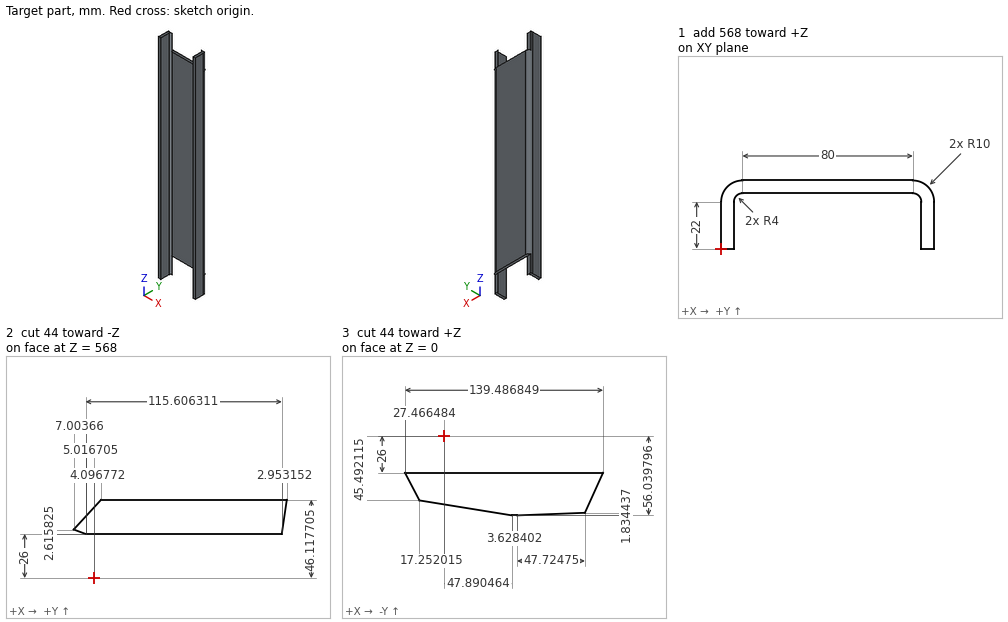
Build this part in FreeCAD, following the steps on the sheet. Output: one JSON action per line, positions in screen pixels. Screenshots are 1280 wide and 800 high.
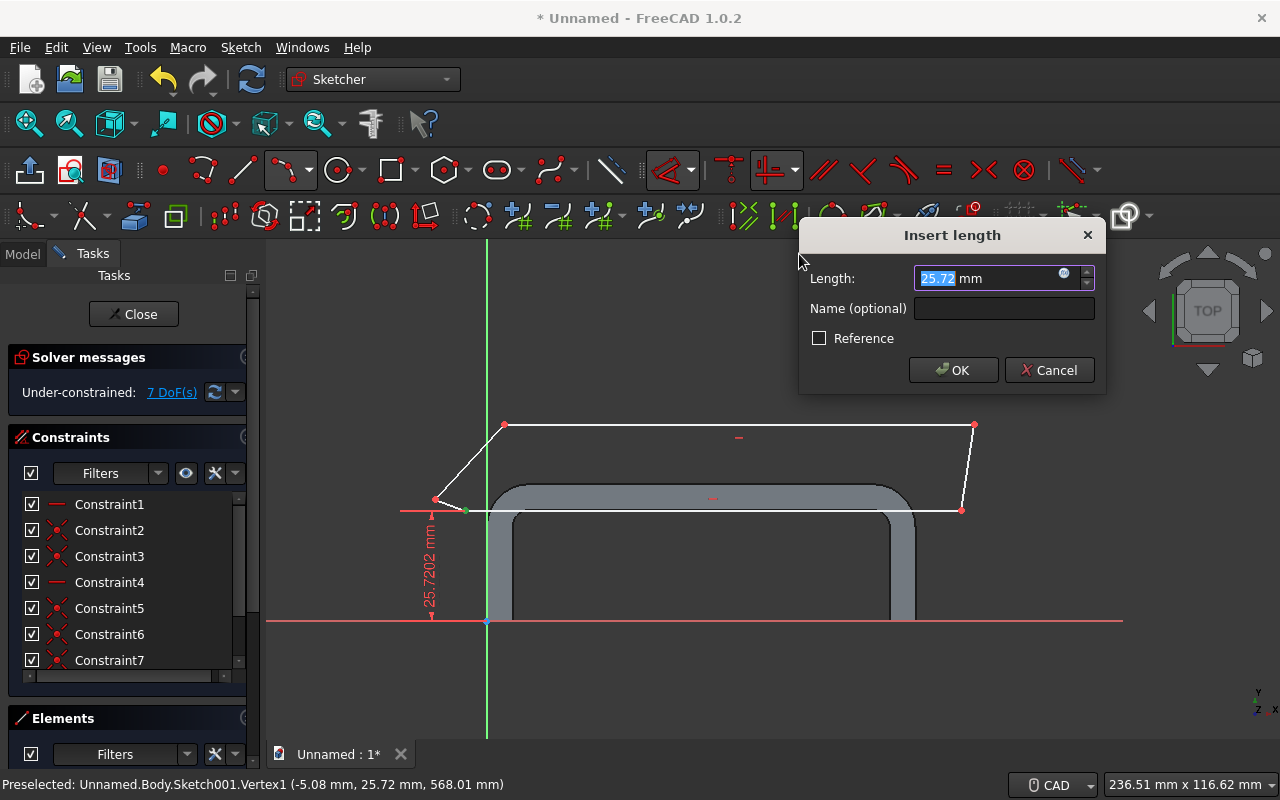
{"action": "type", "text": "26"}
{"action": "key", "text": "Return"}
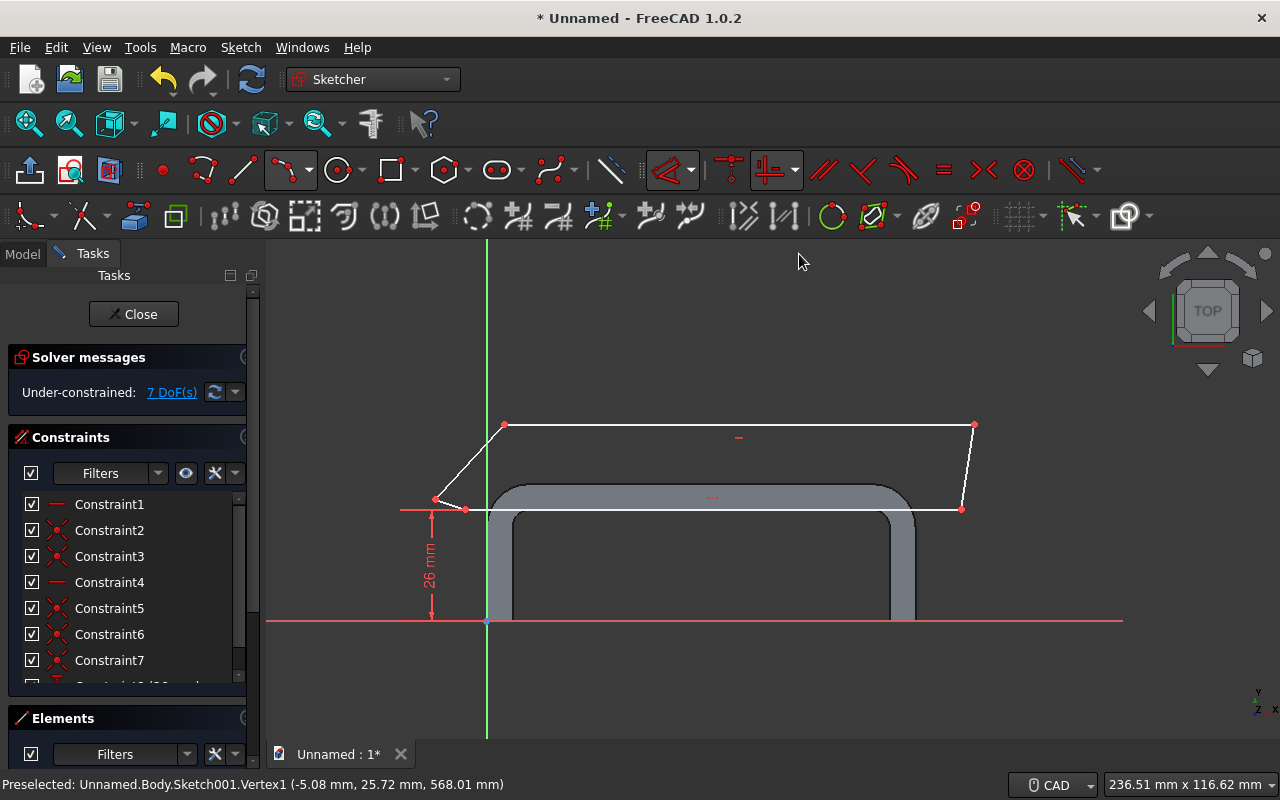
{"action": "scroll", "coordinate": [456, 507], "scroll_direction": "up", "scroll_amount": 2}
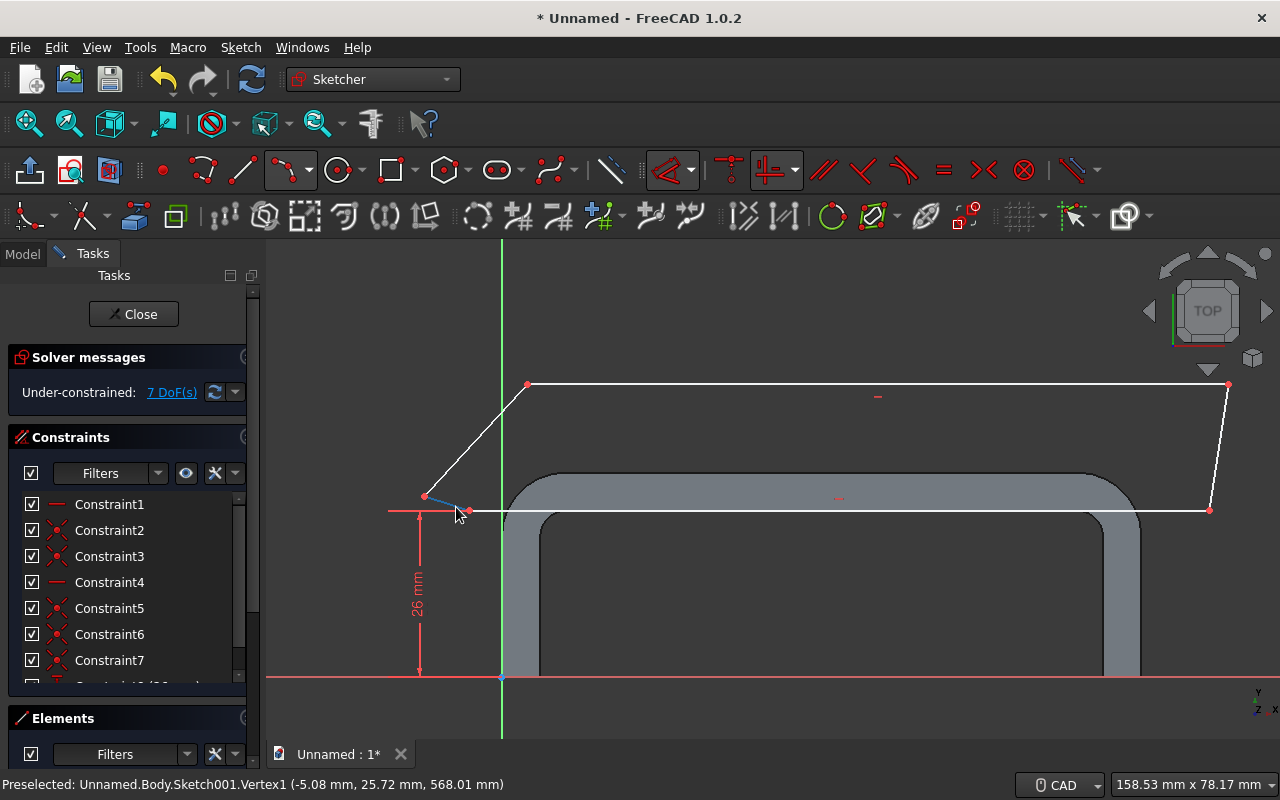
{"action": "left_click", "coordinate": [456, 507]}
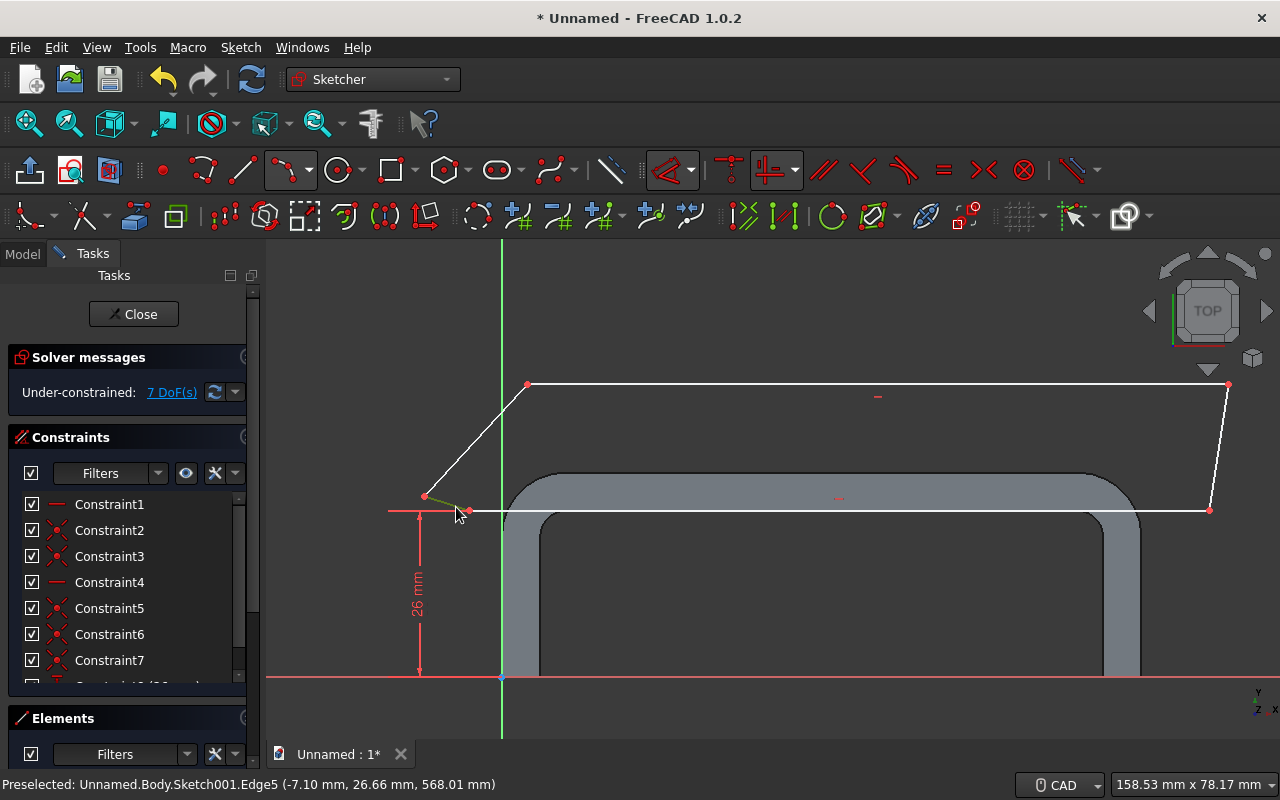
{"action": "left_click", "coordinate": [694, 170]}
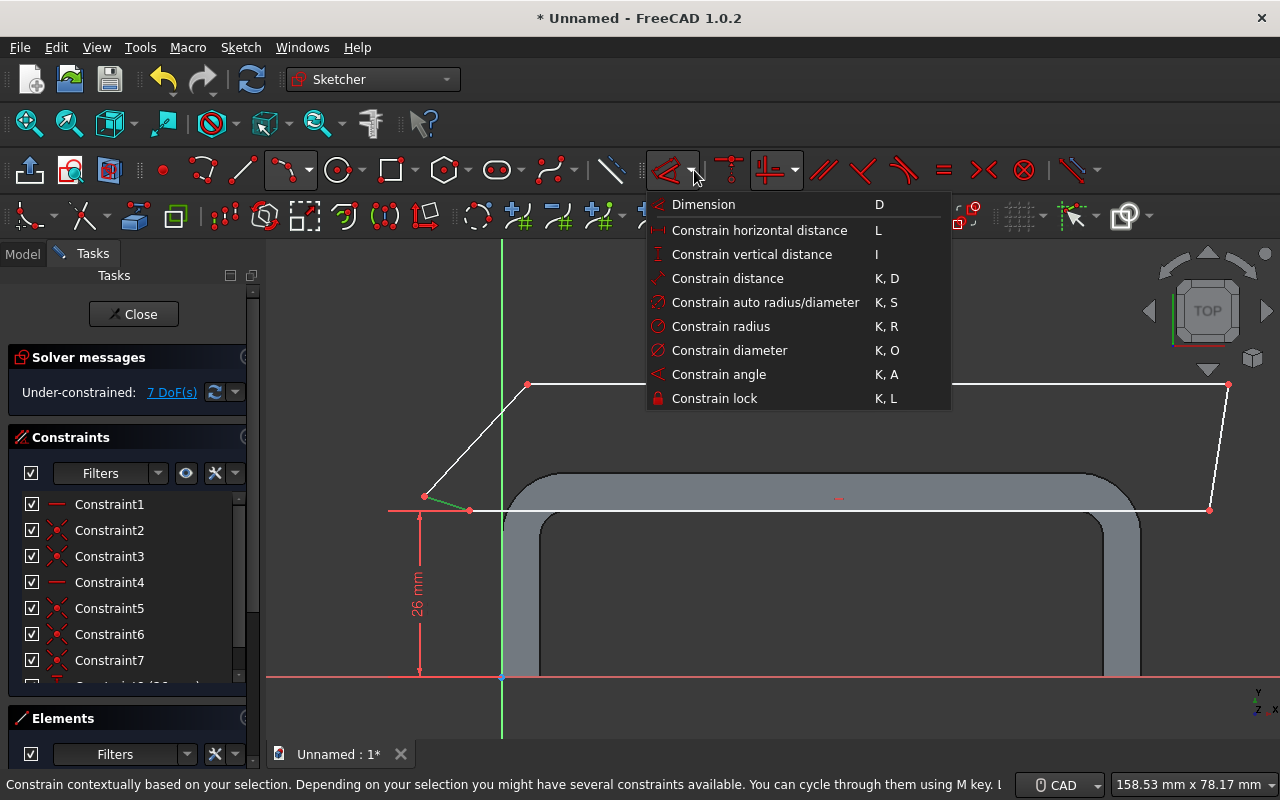
{"action": "left_click", "coordinate": [799, 230]}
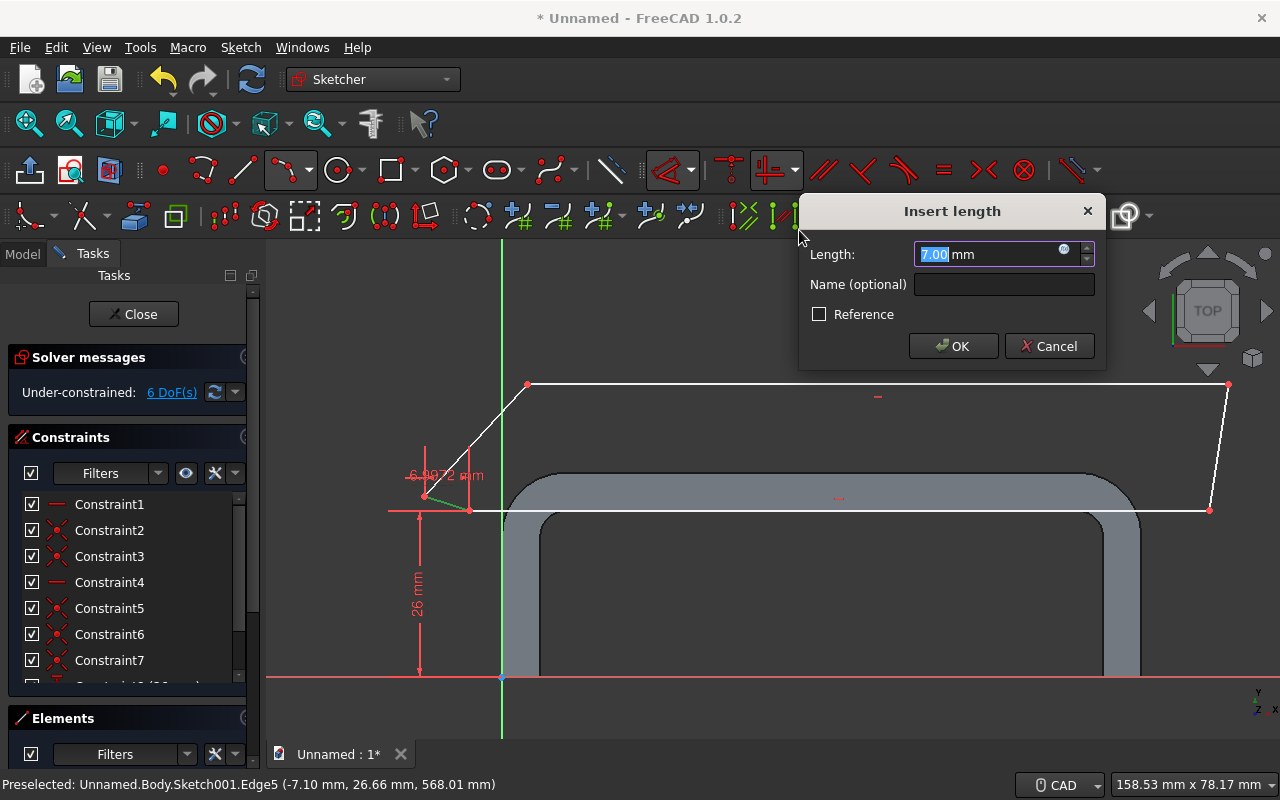
{"action": "type", "text": "7.00366"}
{"action": "key", "text": "Return"}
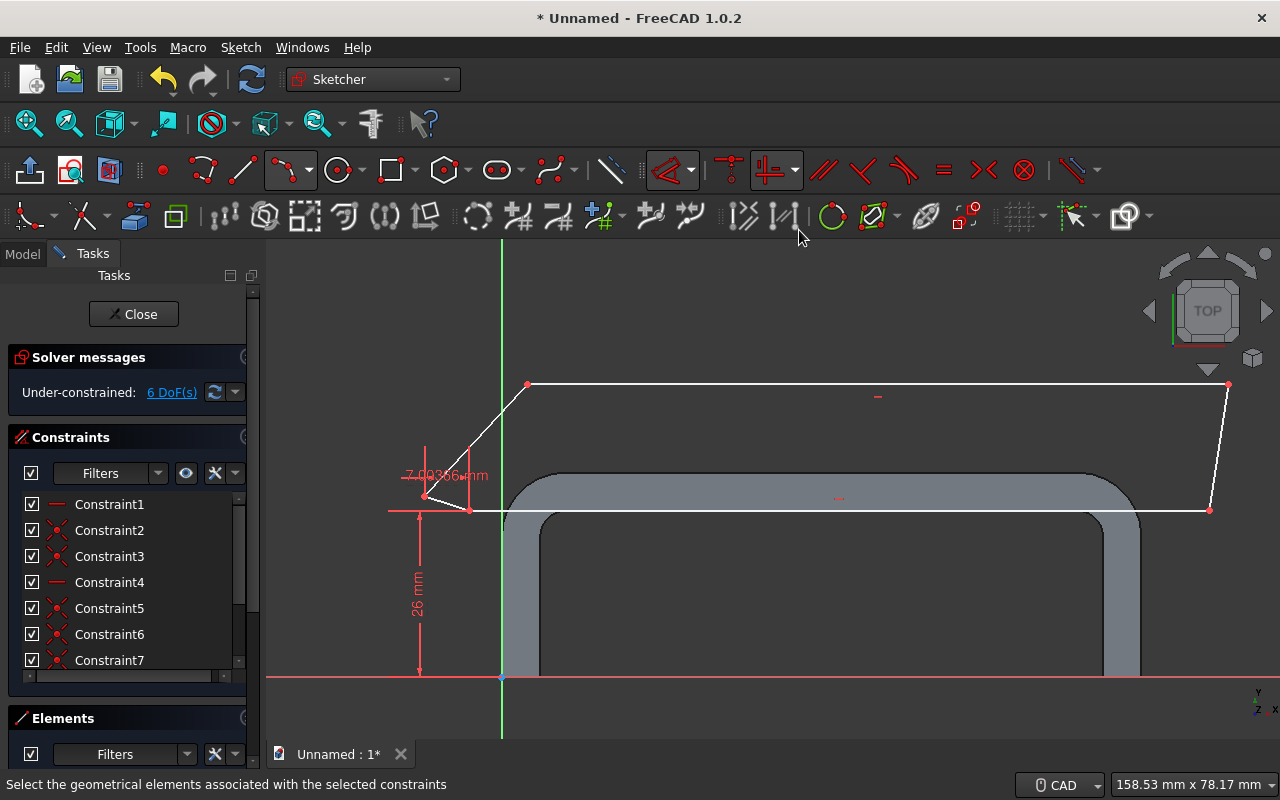
{"action": "scroll", "coordinate": [469, 511], "scroll_direction": "up", "scroll_amount": 2}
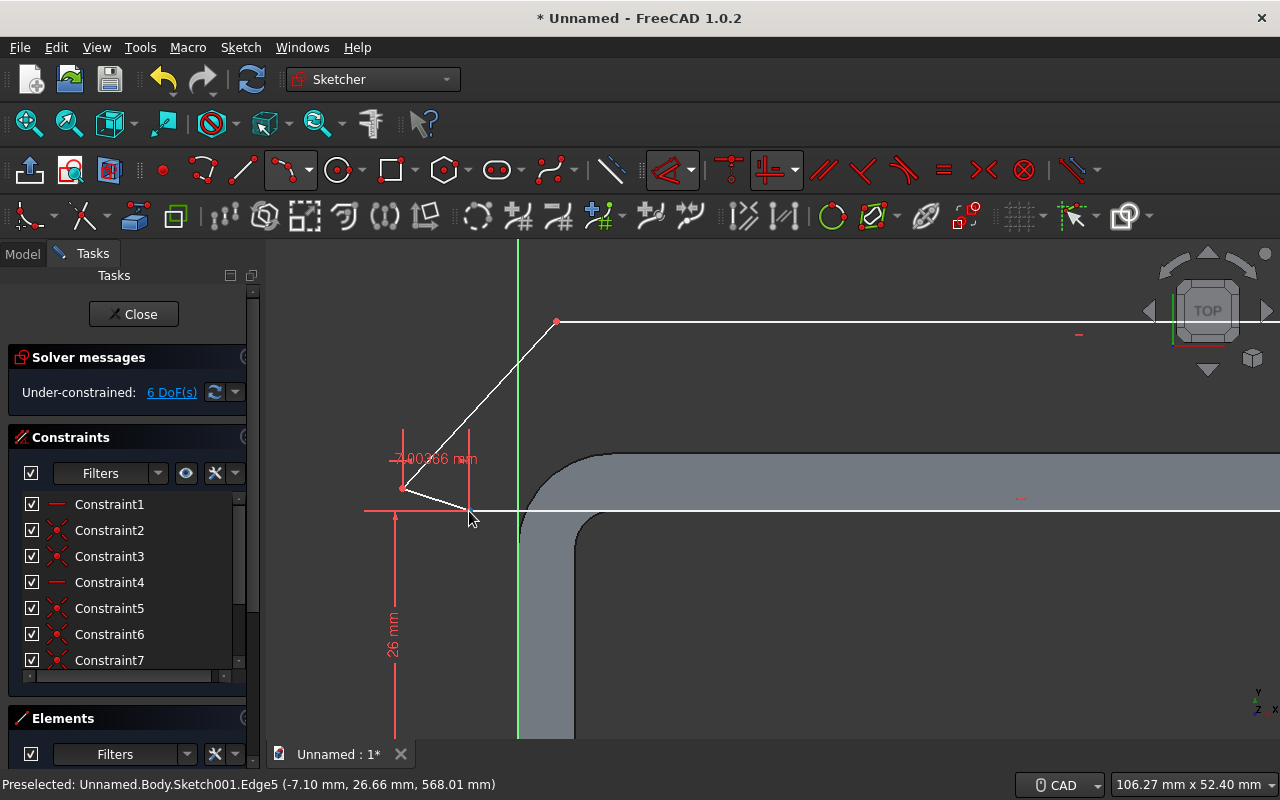
{"action": "left_click", "coordinate": [469, 511]}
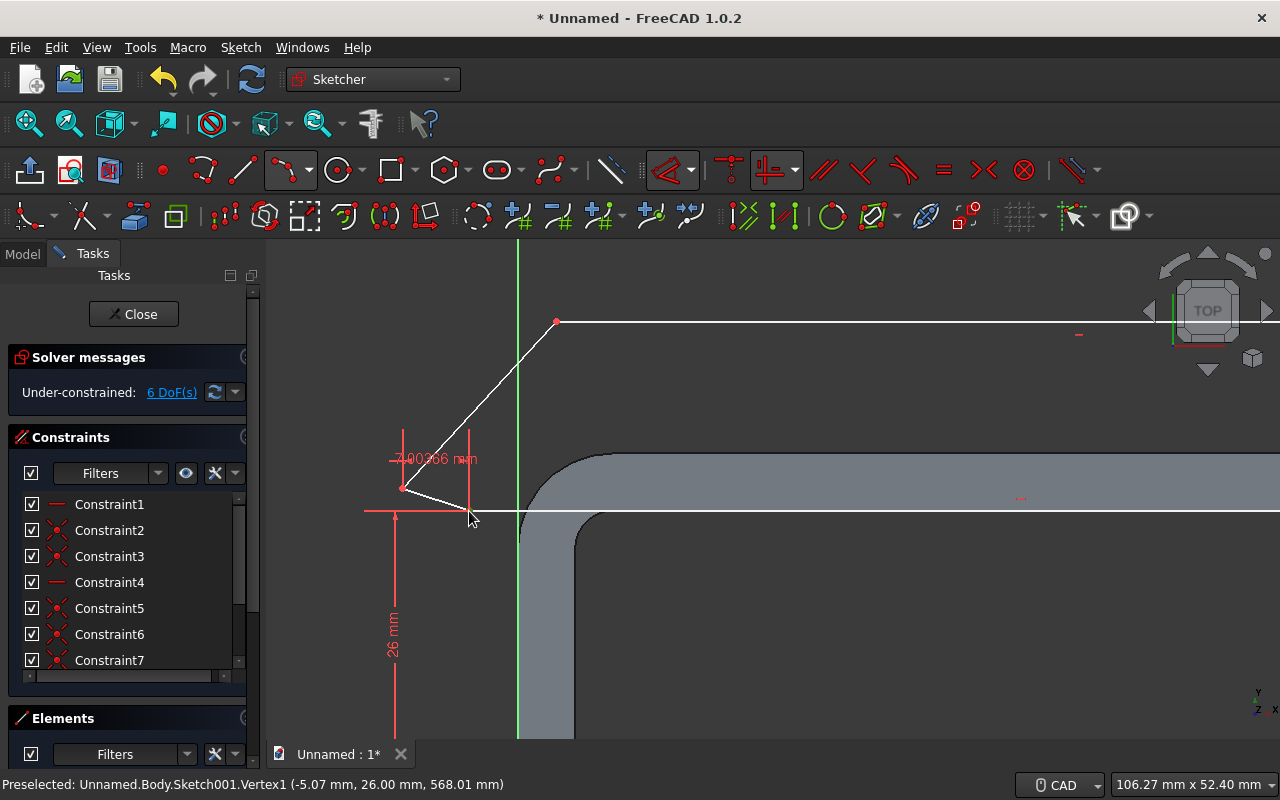
{"action": "left_click", "coordinate": [694, 170]}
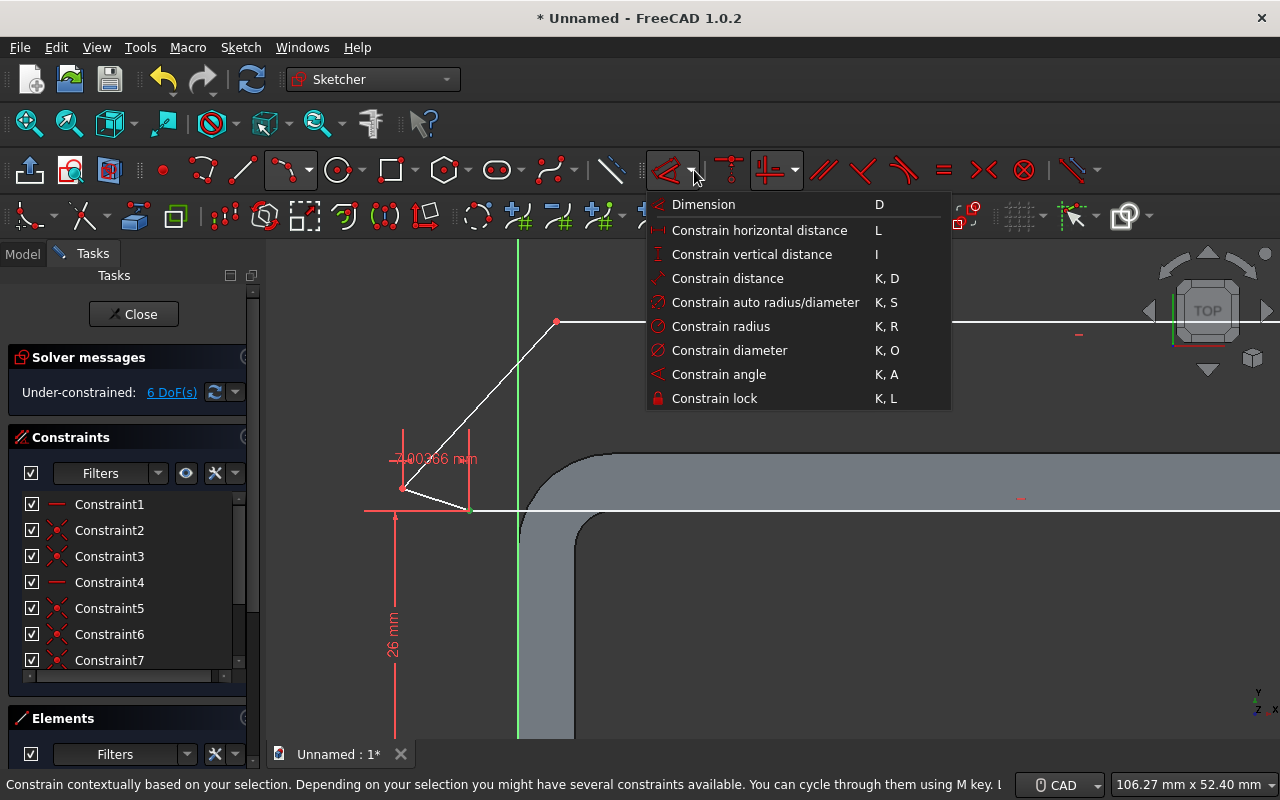
{"action": "left_click", "coordinate": [799, 230]}